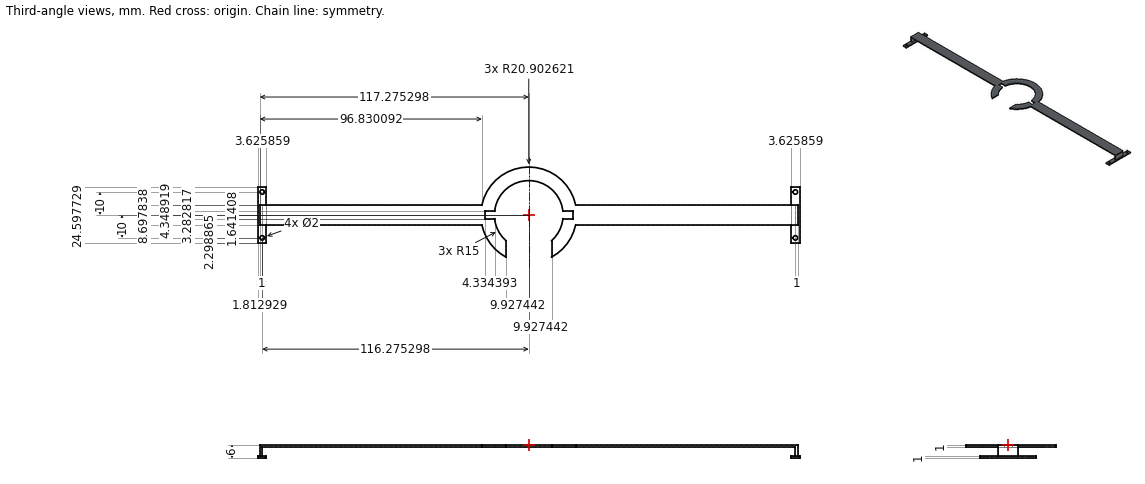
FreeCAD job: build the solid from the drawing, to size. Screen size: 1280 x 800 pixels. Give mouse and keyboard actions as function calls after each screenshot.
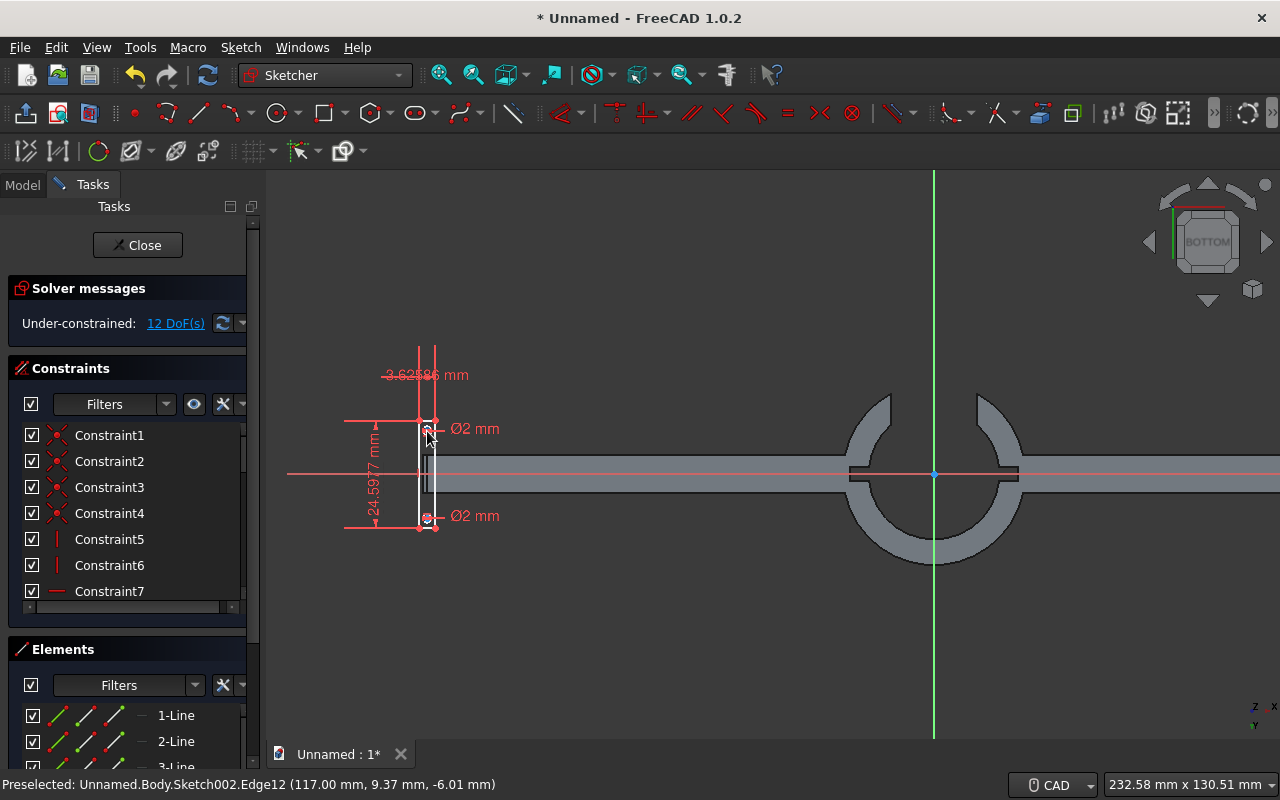
click(427, 431)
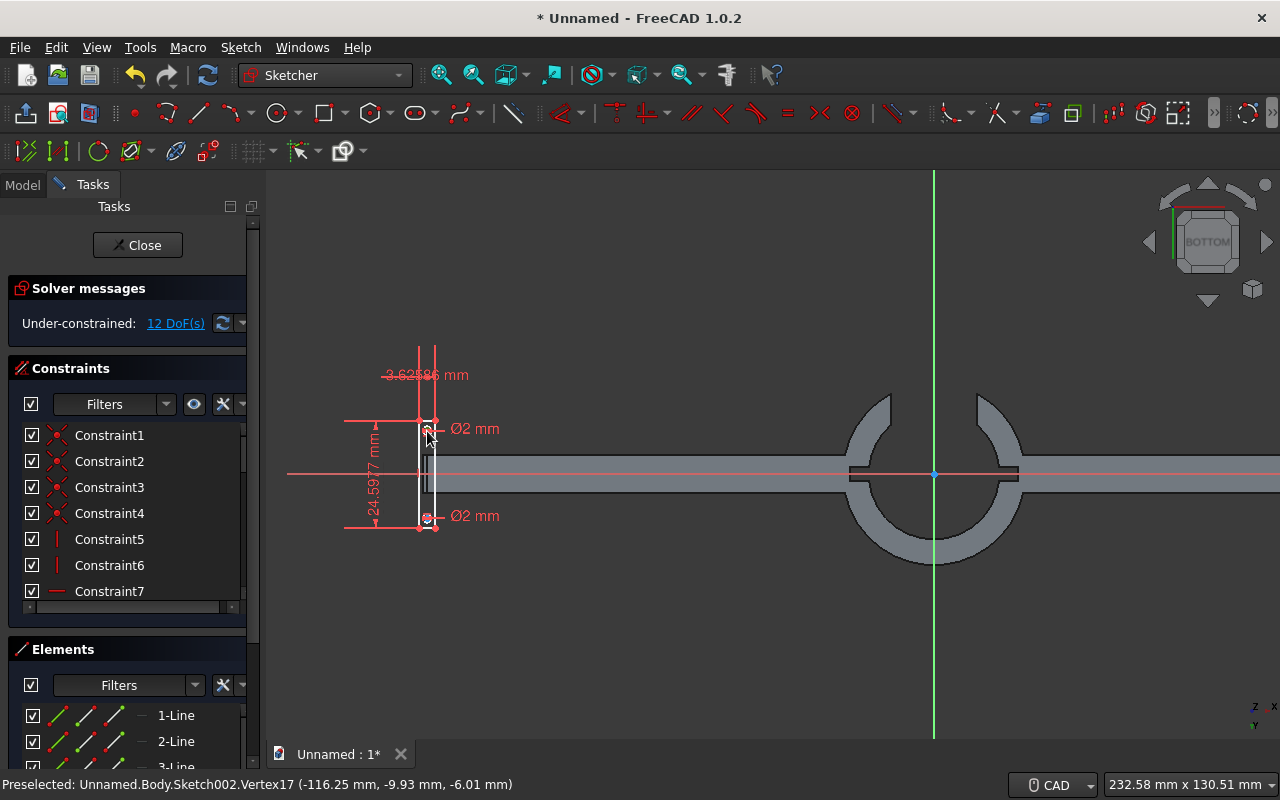
click(427, 518)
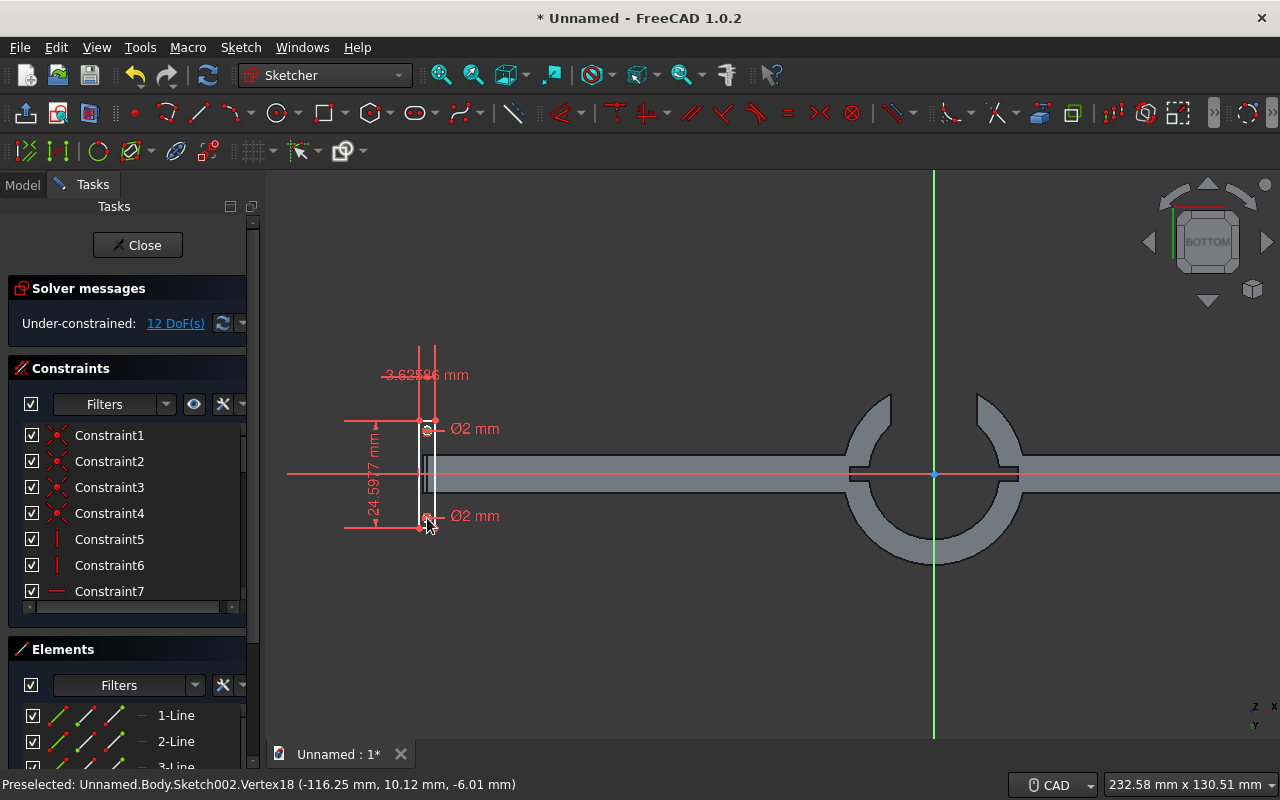
key(v)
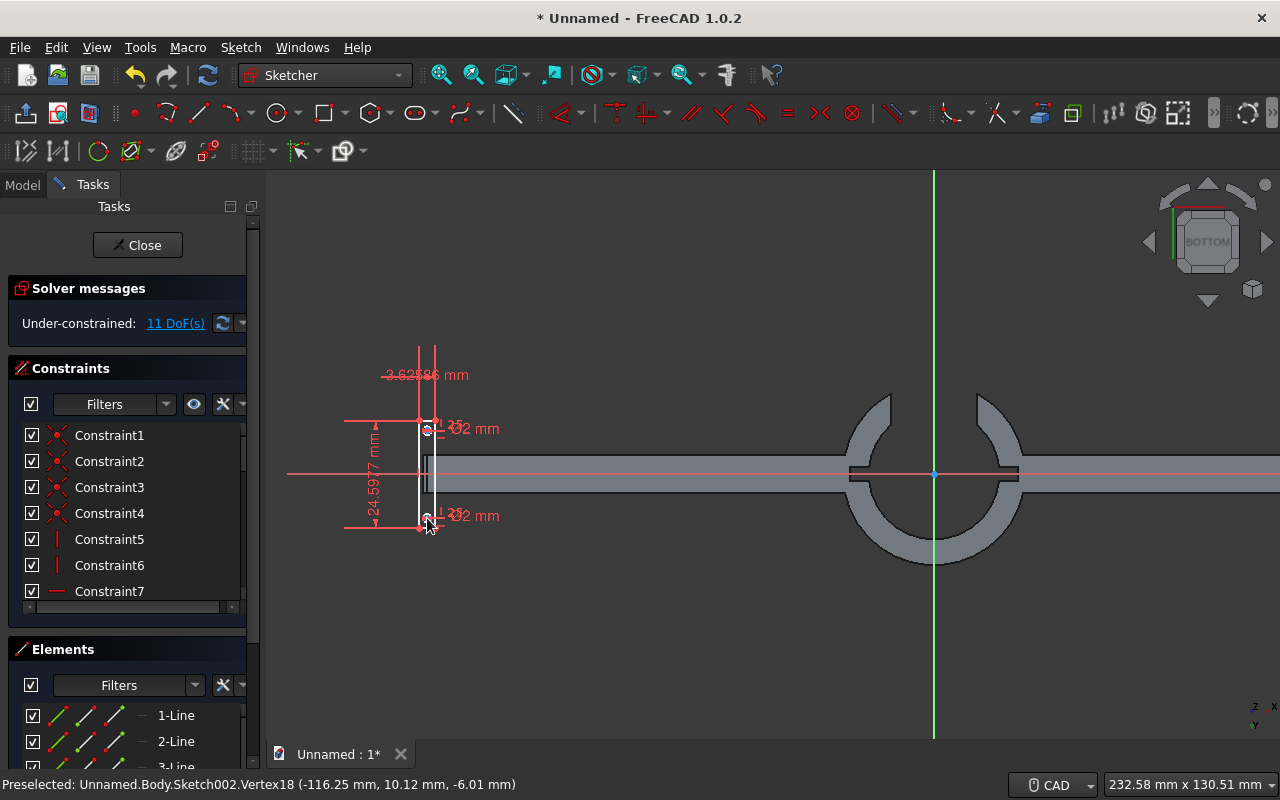
scroll(425, 431, down, 3)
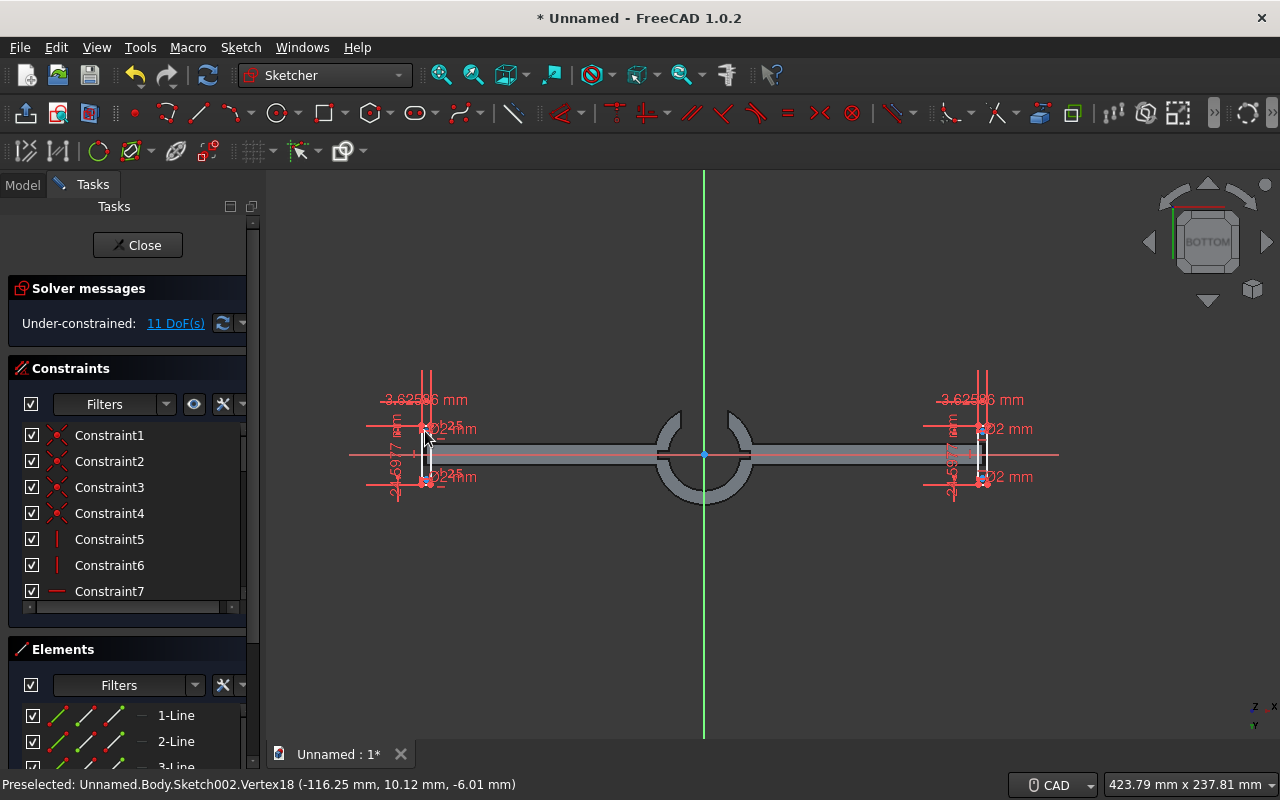
scroll(983, 431, up, 3)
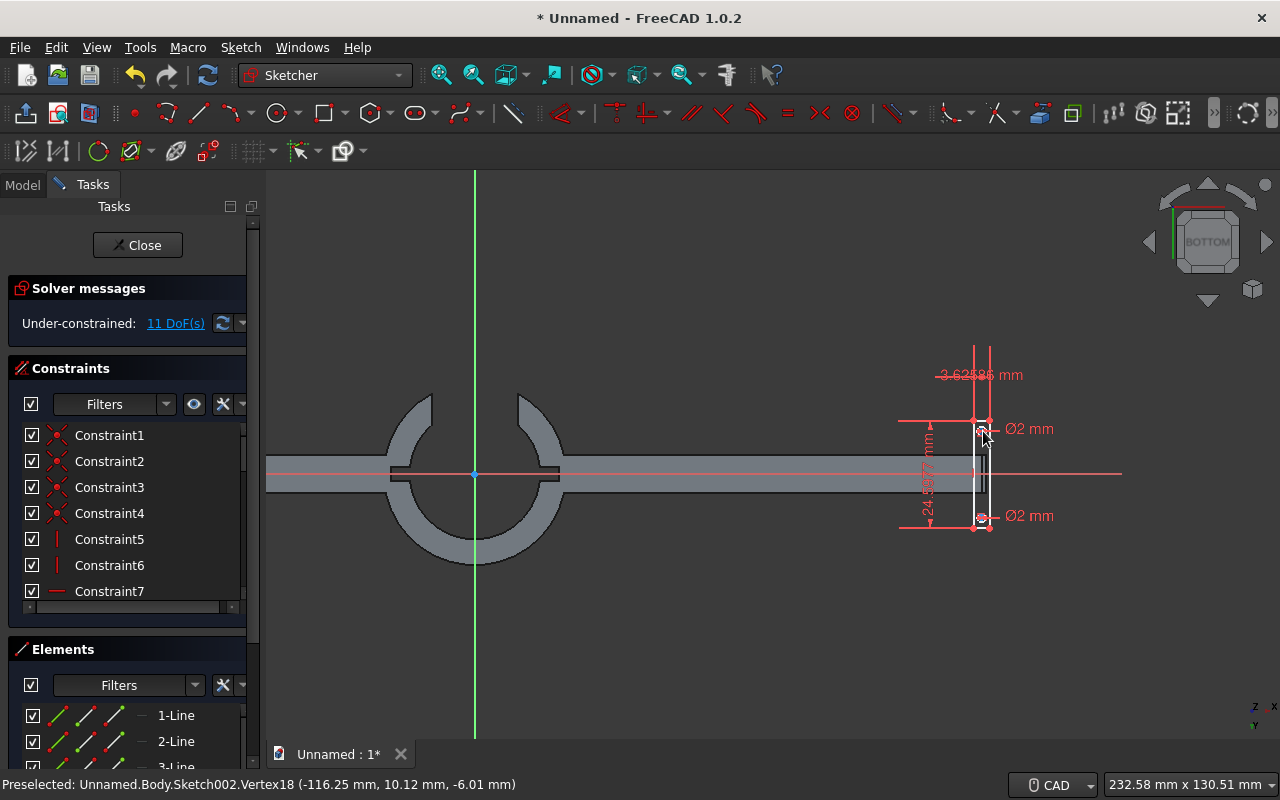
click(982, 431)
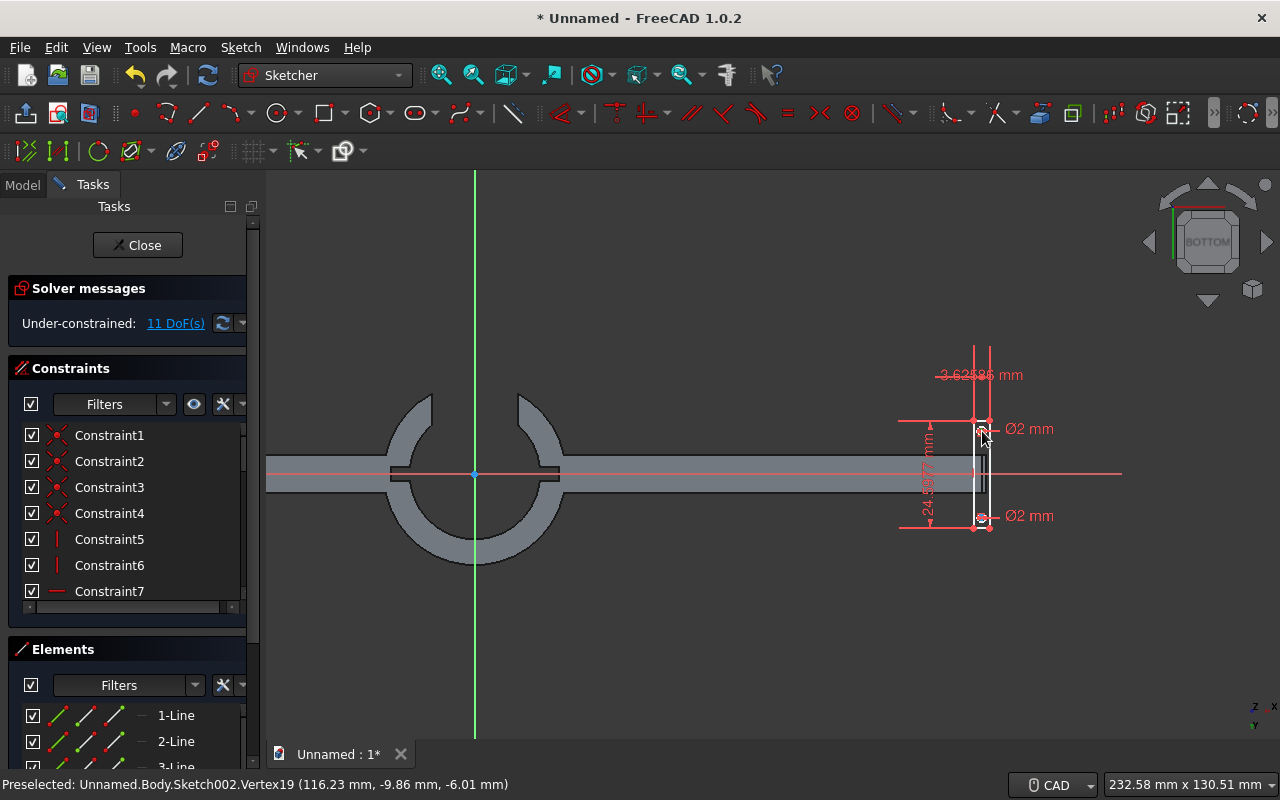
click(982, 518)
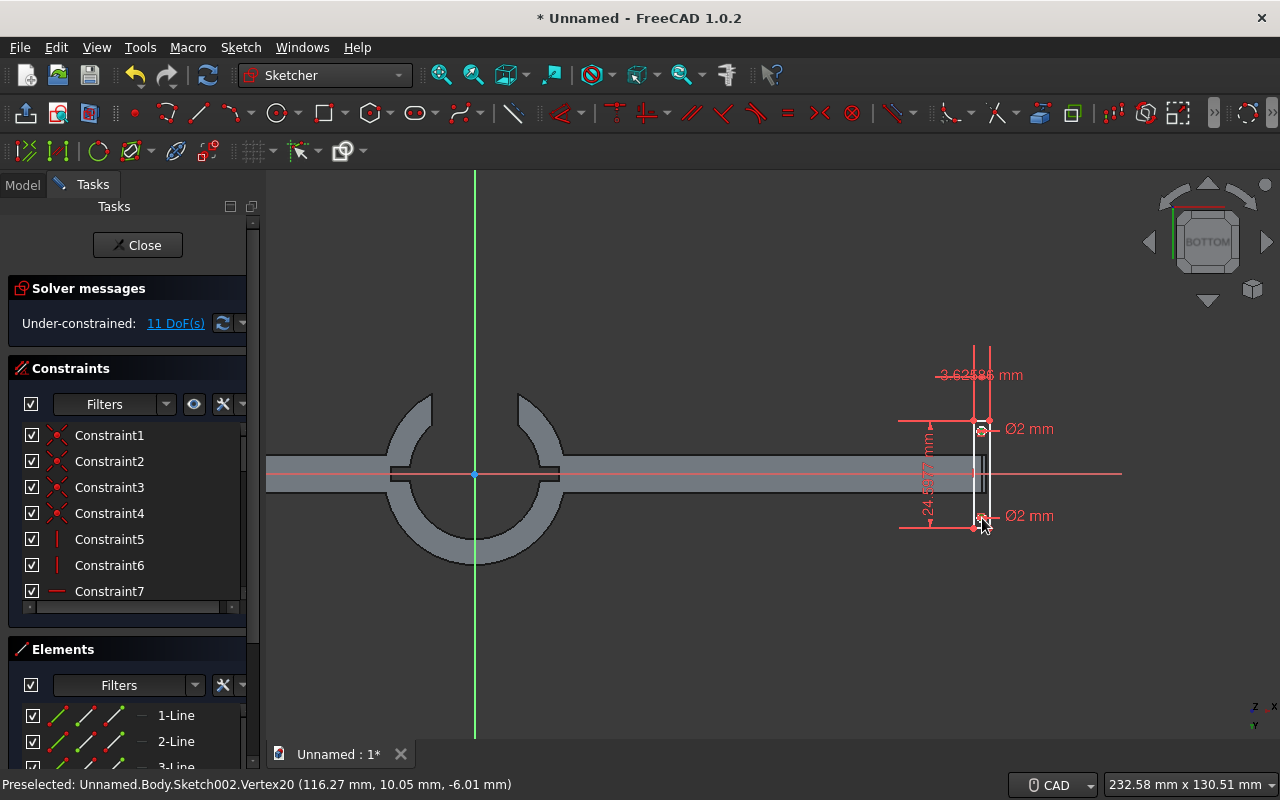
key(v)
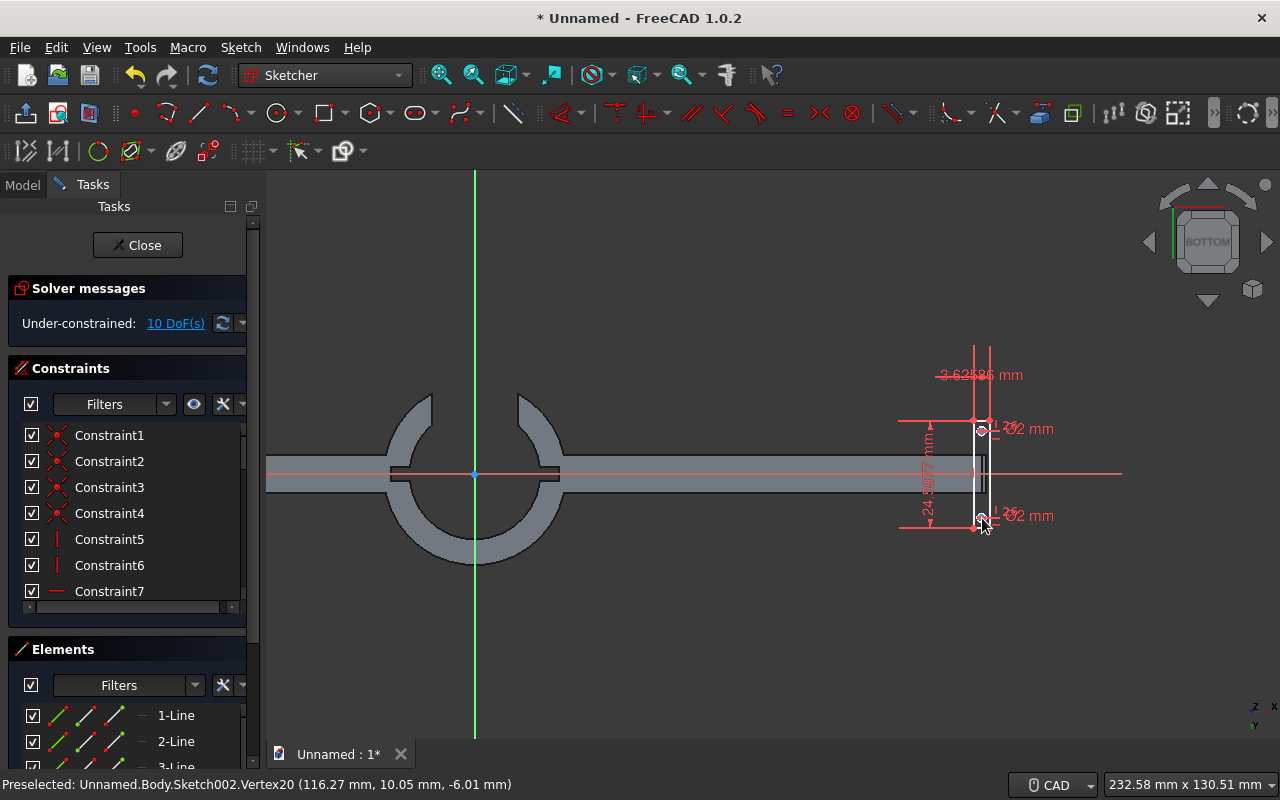
scroll(984, 431, down, 3)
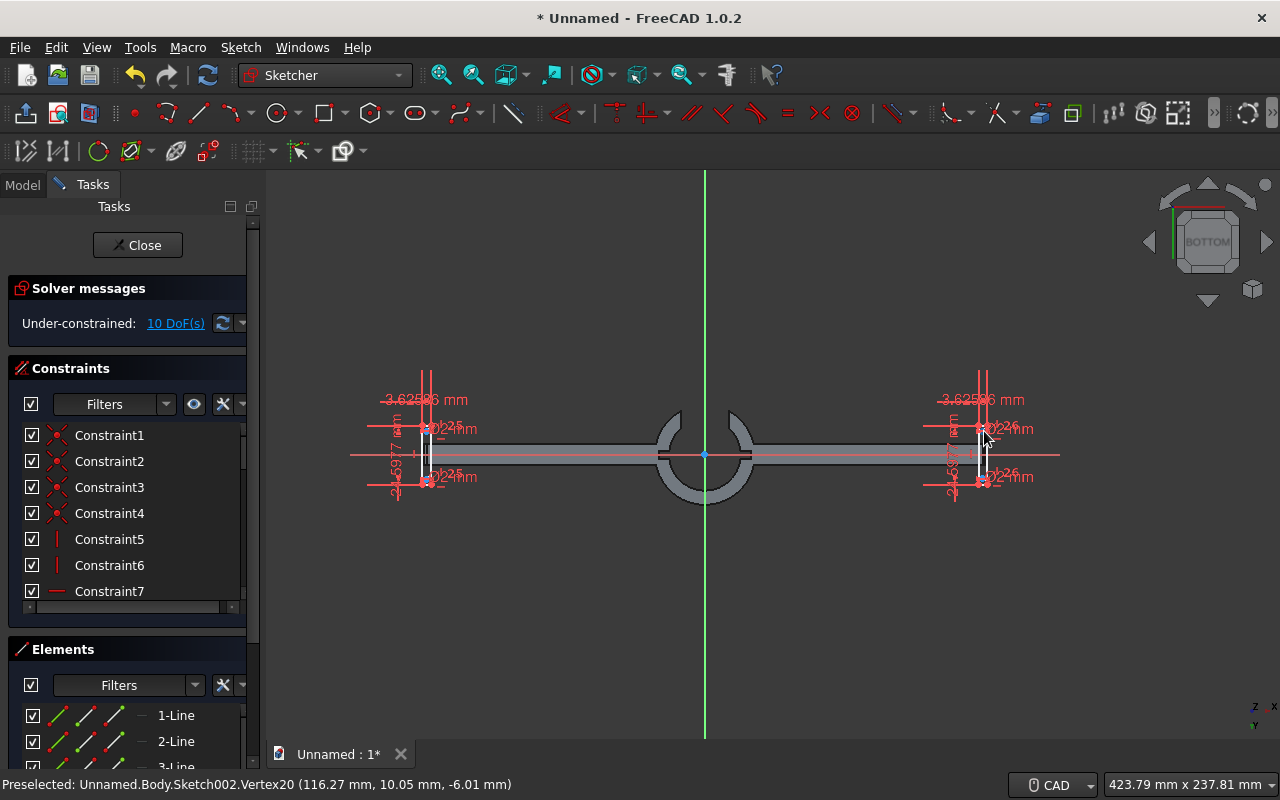
scroll(427, 431, up, 3)